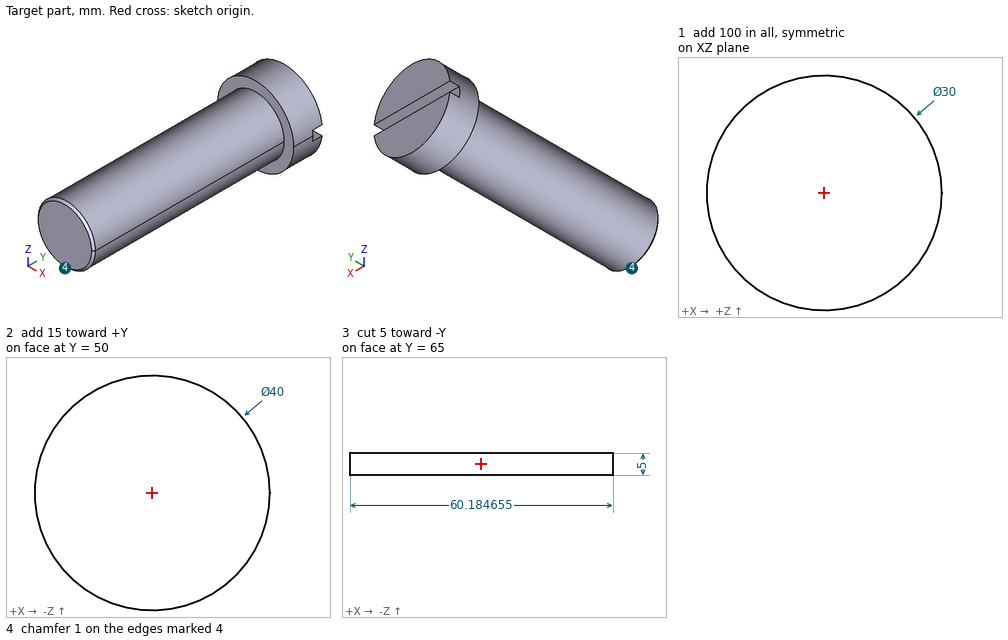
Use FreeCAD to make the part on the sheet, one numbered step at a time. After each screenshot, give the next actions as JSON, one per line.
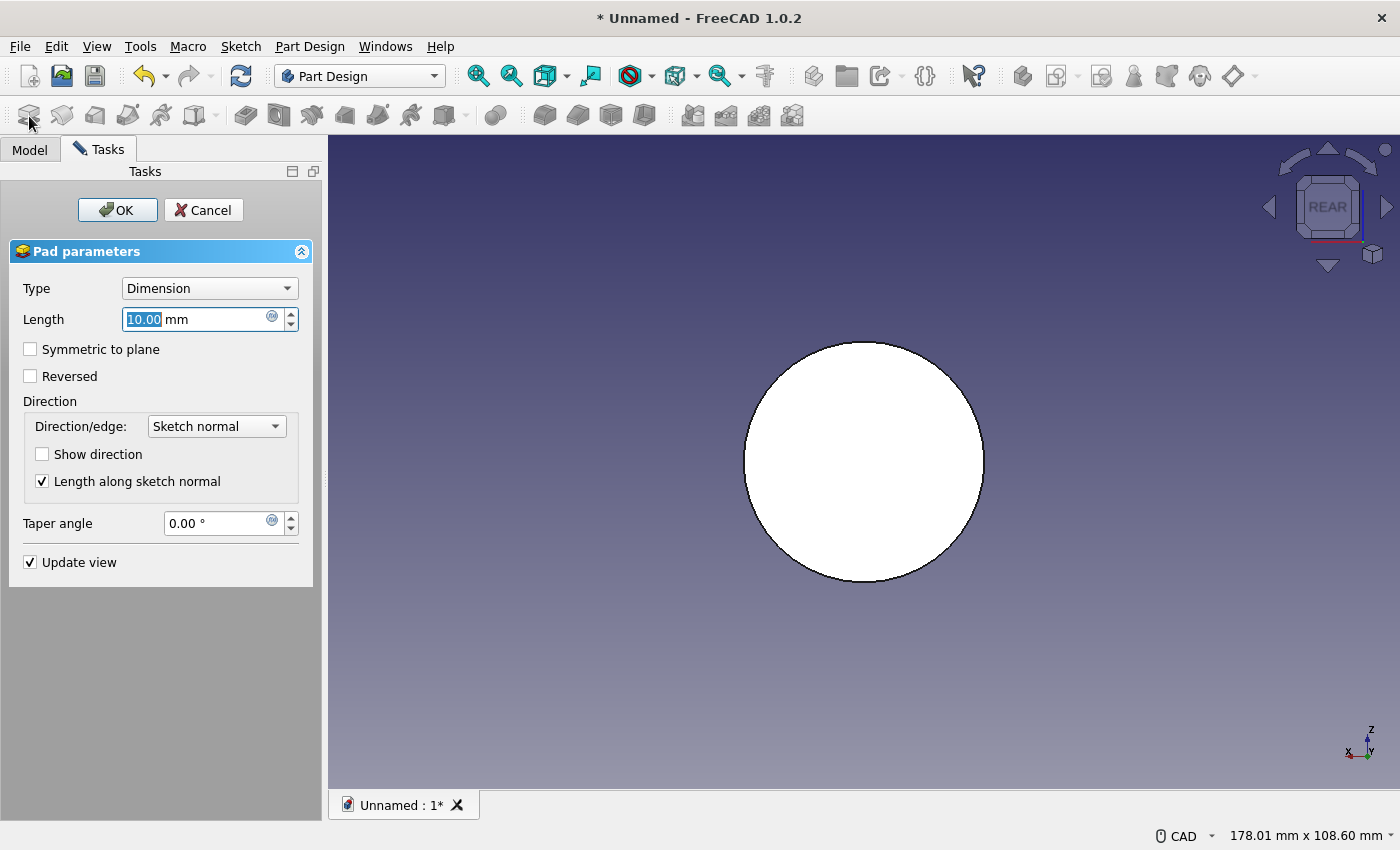
{"action": "type", "text": "15"}
{"action": "key", "text": "Tab"}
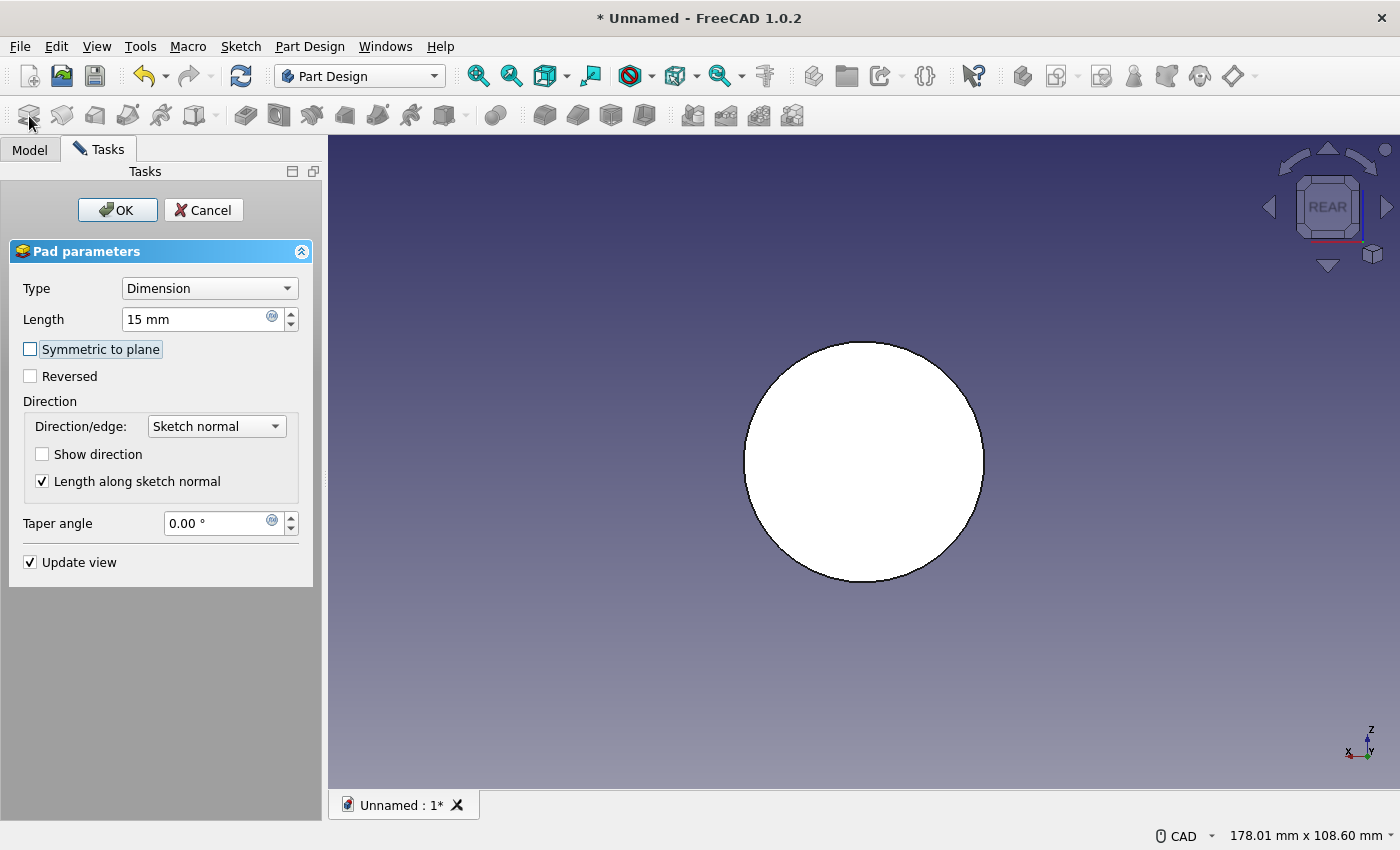
{"action": "left_click", "coordinate": [118, 210]}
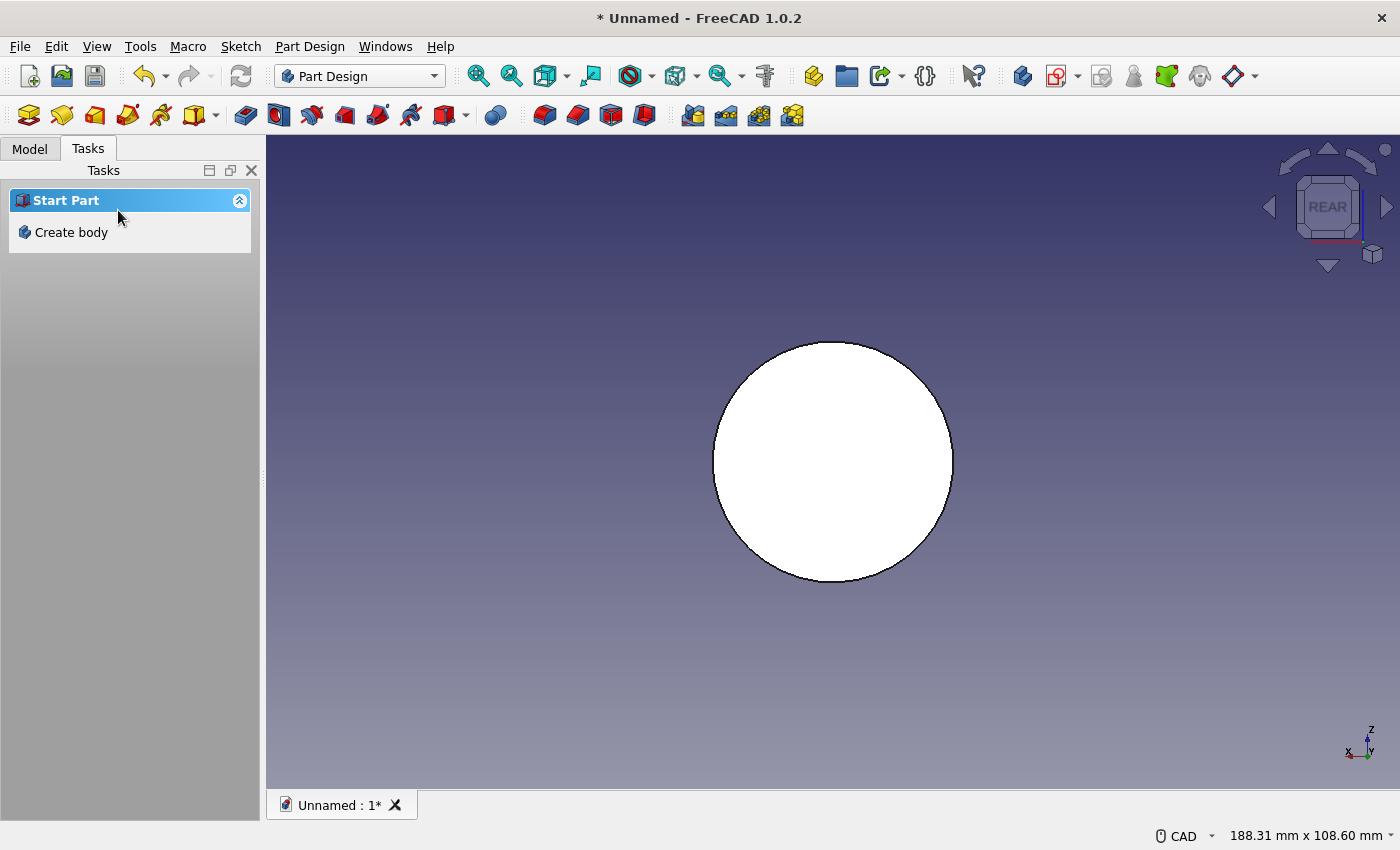
{"action": "left_click", "coordinate": [479, 76]}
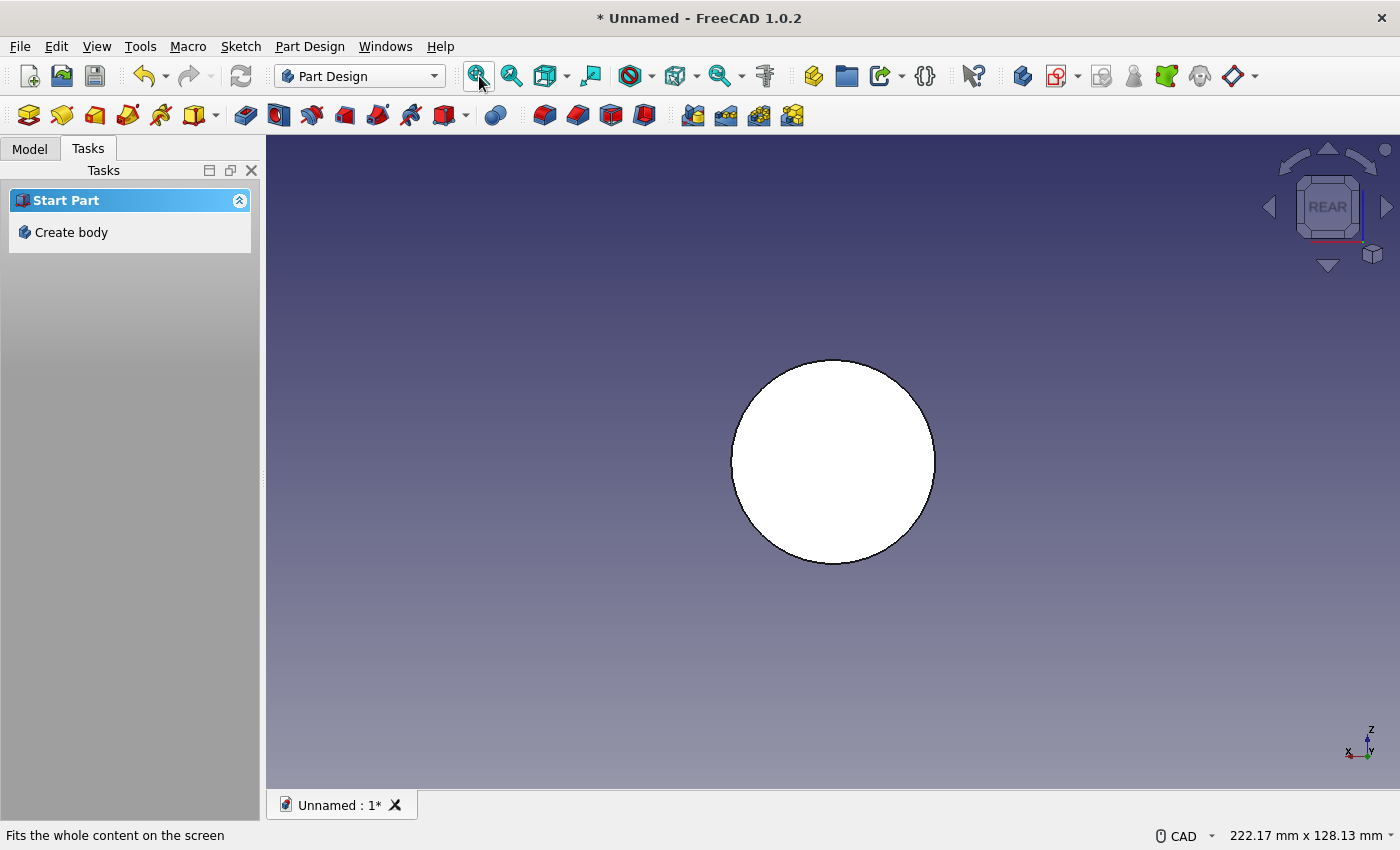
{"action": "left_click", "coordinate": [833, 461]}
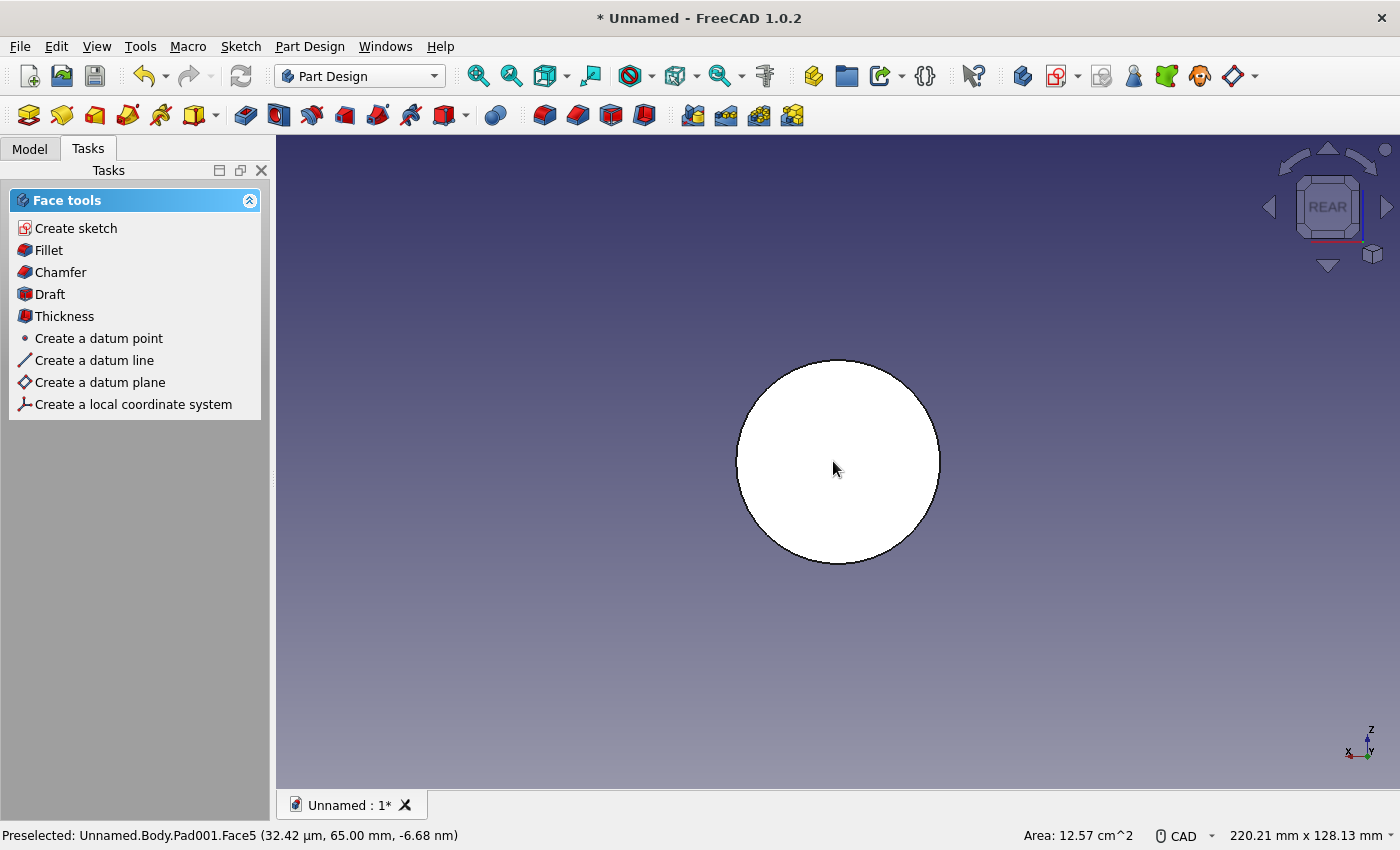
{"action": "left_click", "coordinate": [1056, 76]}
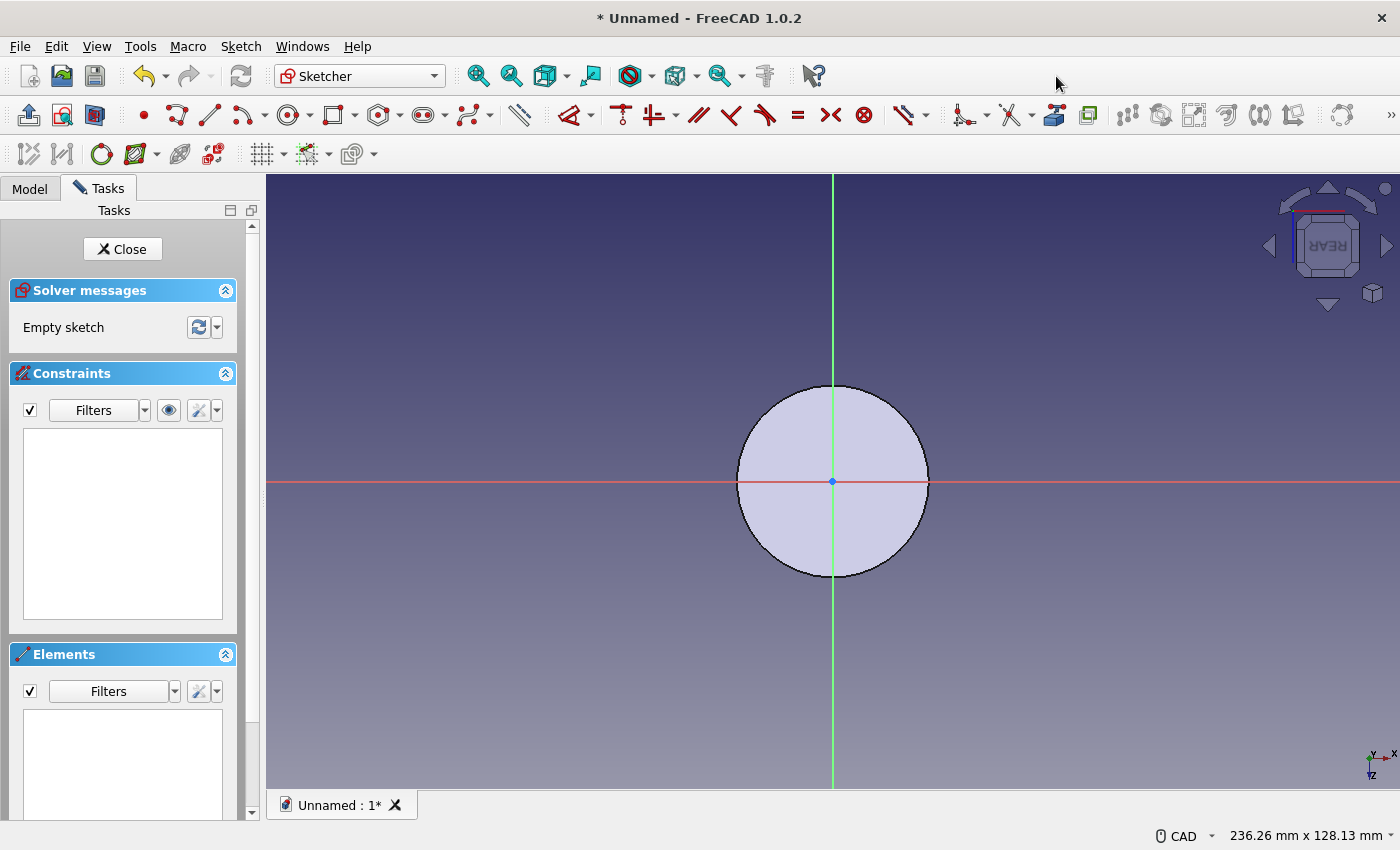
{"action": "scroll", "coordinate": [889, 481], "scroll_direction": "up", "scroll_amount": 4}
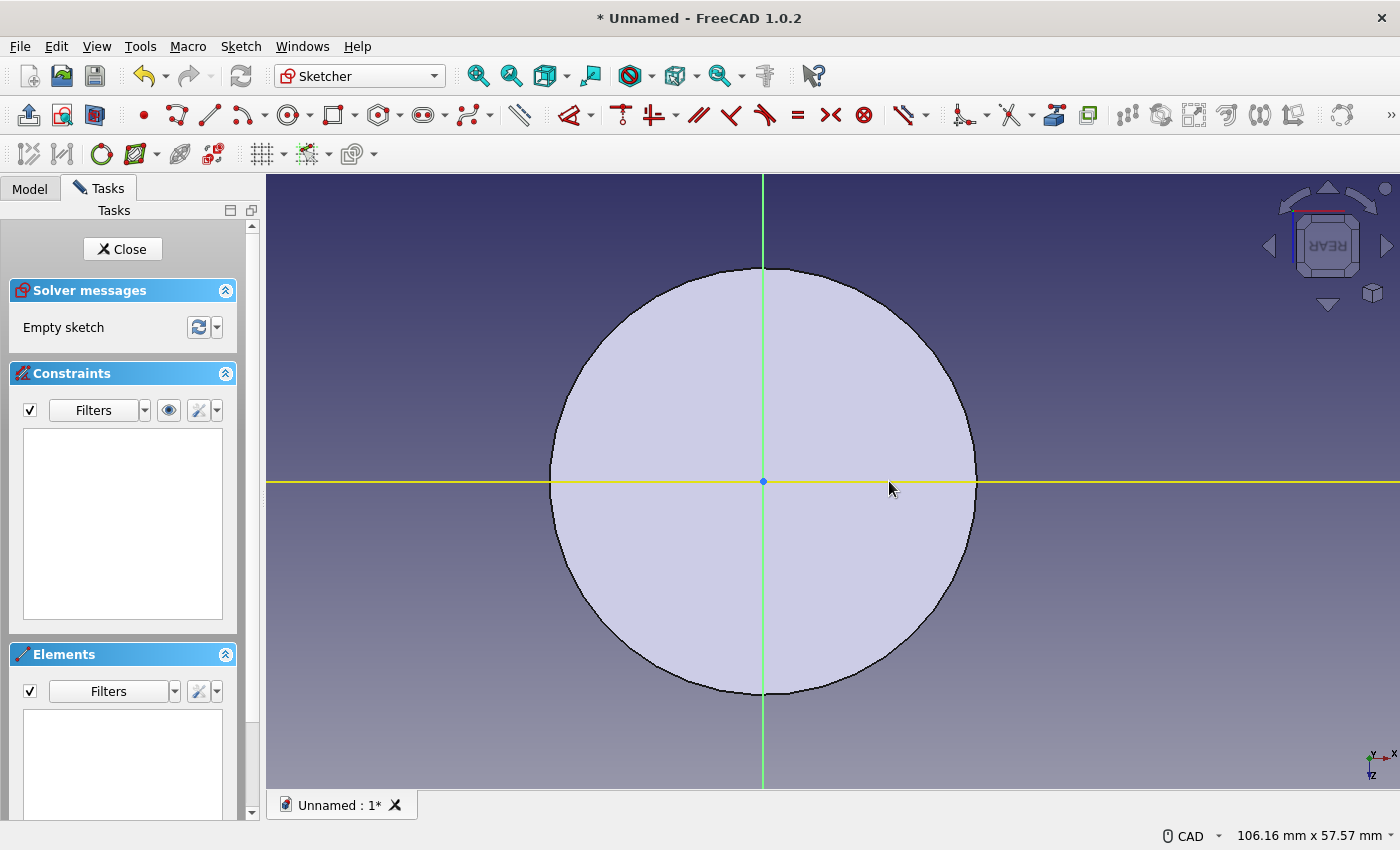
{"action": "left_click", "coordinate": [354, 116]}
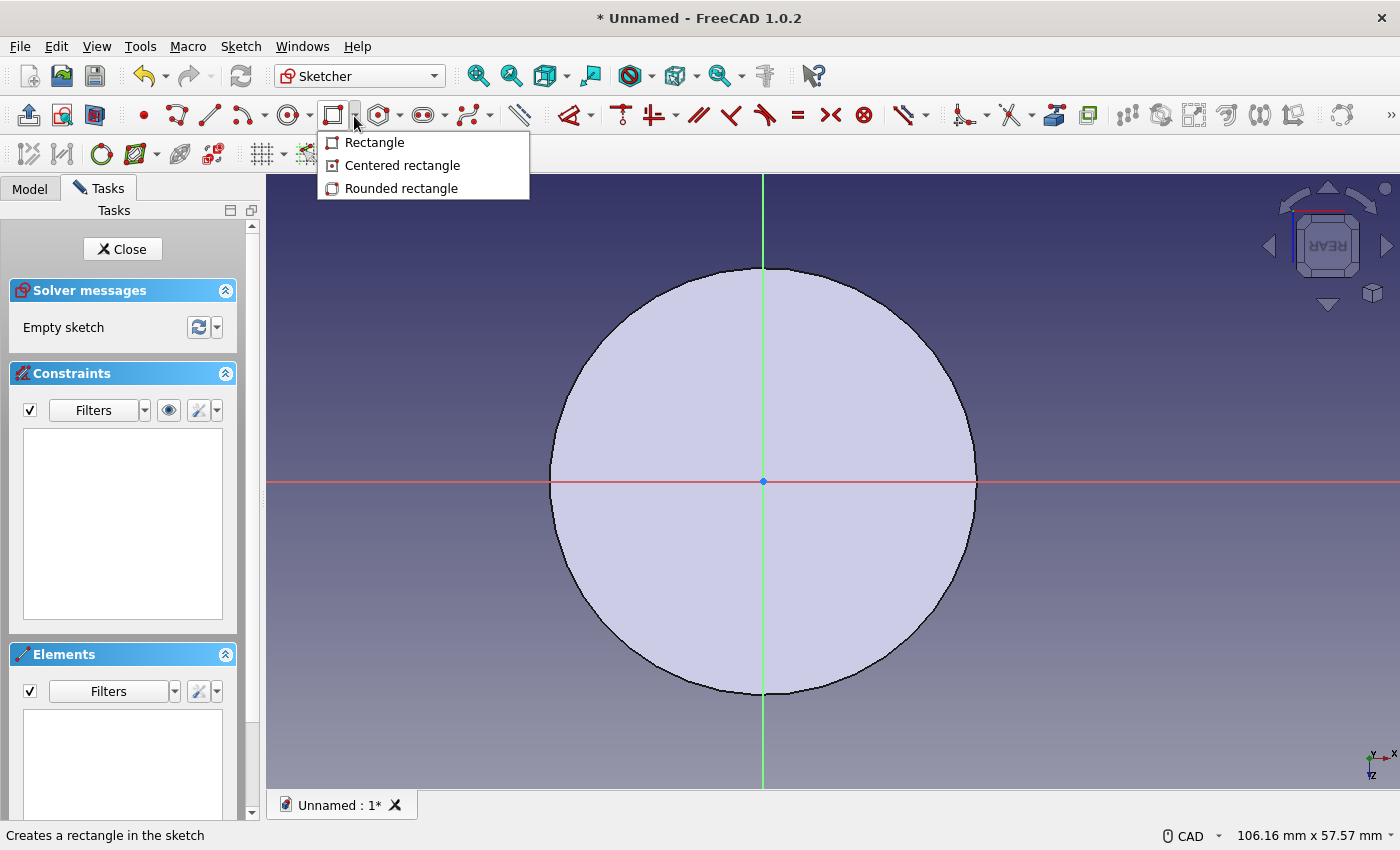
{"action": "left_click", "coordinate": [424, 166]}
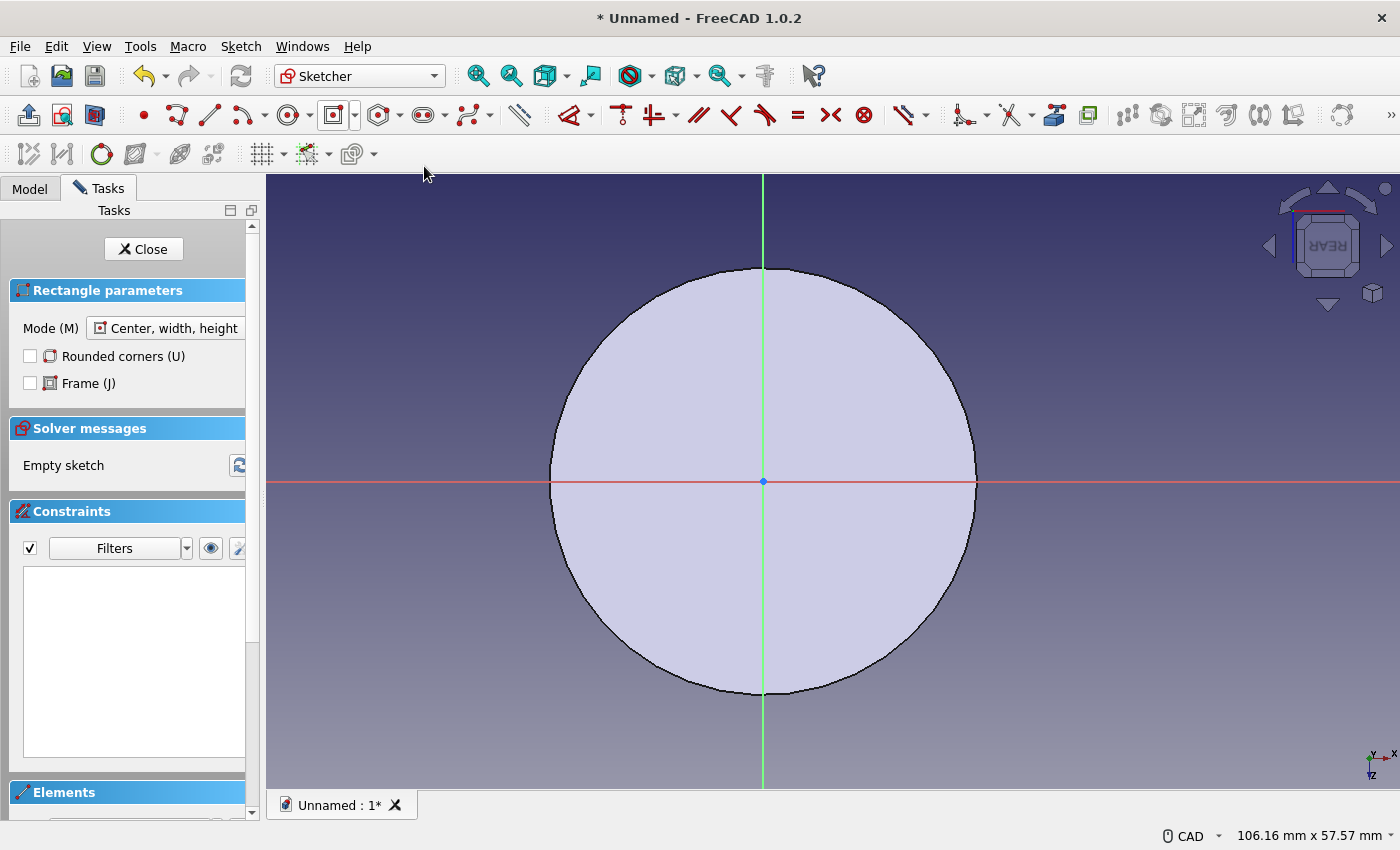
{"action": "left_click", "coordinate": [763, 481]}
{"action": "left_click", "coordinate": [1085, 455]}
{"action": "key", "text": "Escape"}